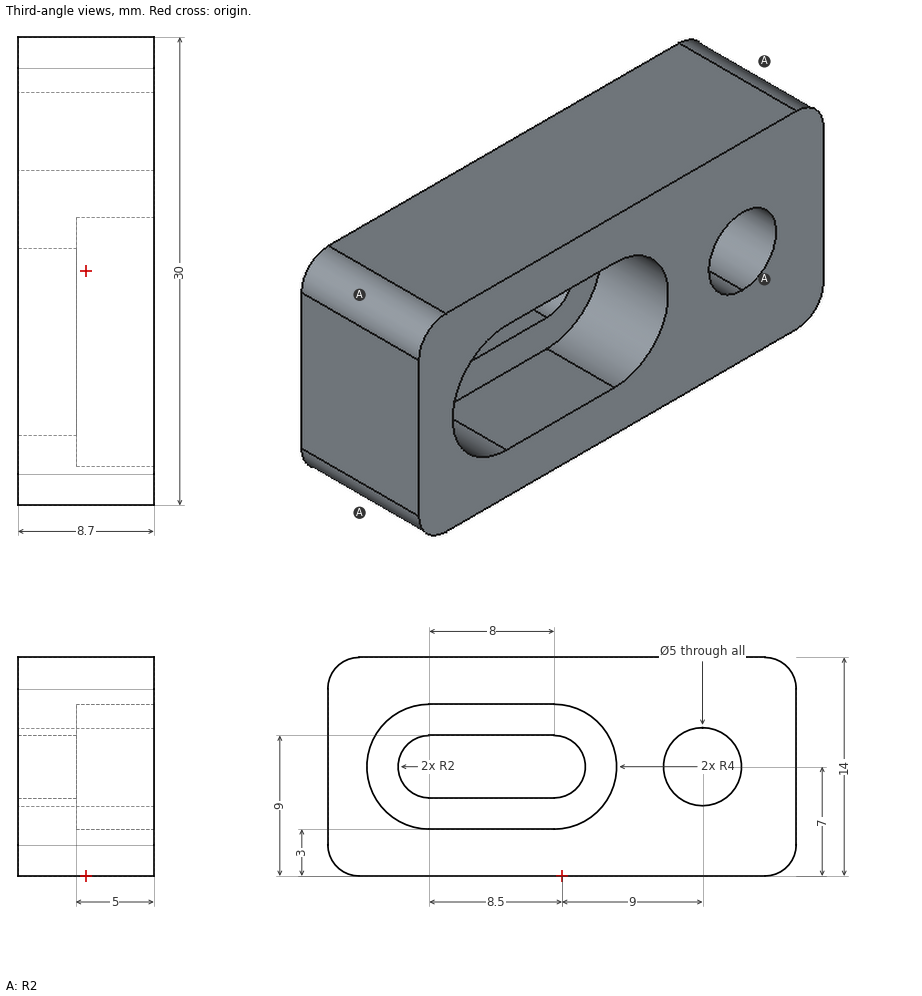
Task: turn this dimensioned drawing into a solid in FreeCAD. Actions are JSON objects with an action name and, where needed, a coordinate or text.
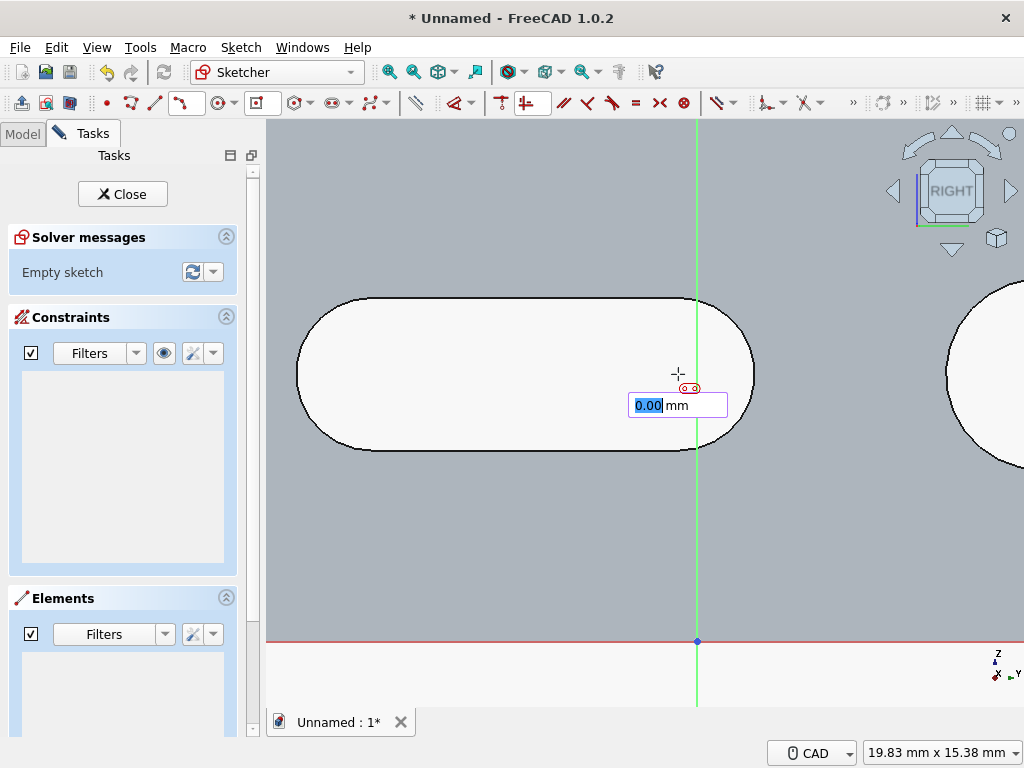
{"action": "left_click", "coordinate": [525, 527]}
{"action": "key", "text": "Escape"}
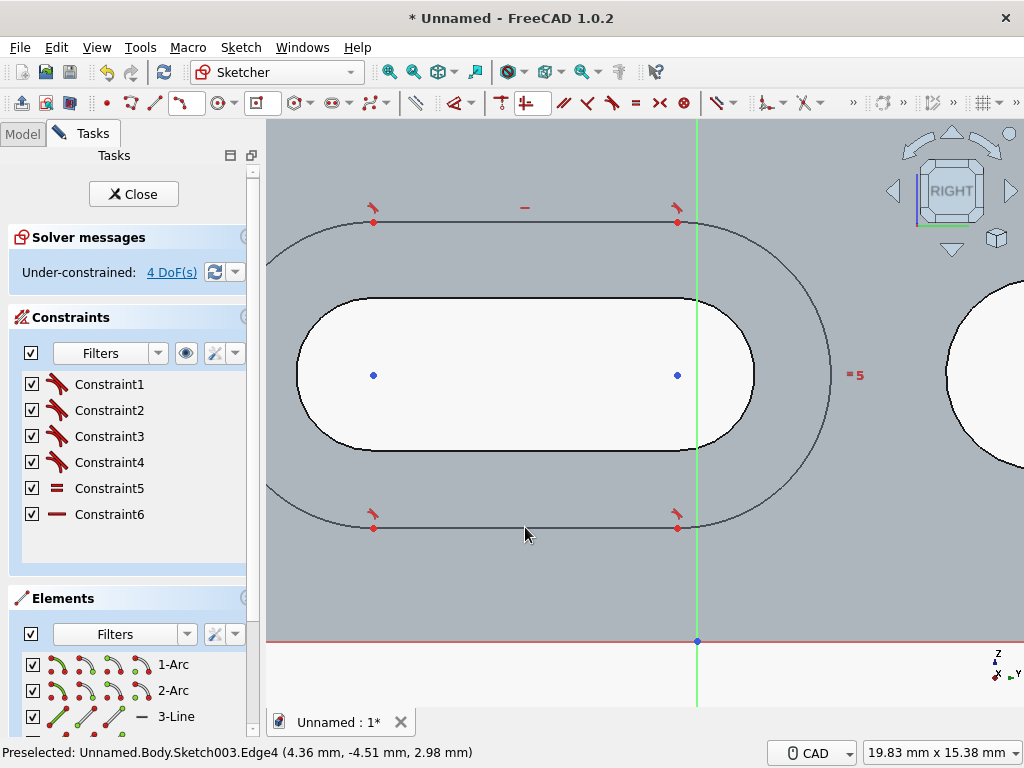
{"action": "left_click", "coordinate": [454, 104]}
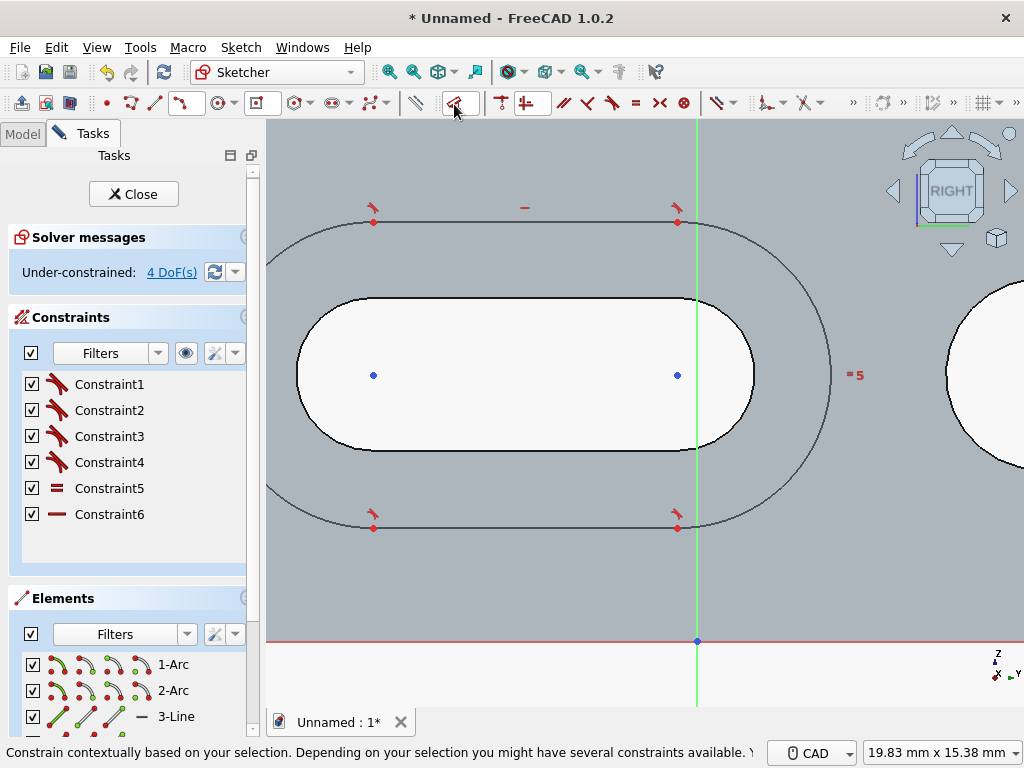
{"action": "scroll", "coordinate": [680, 375], "scroll_direction": "down", "scroll_amount": 2}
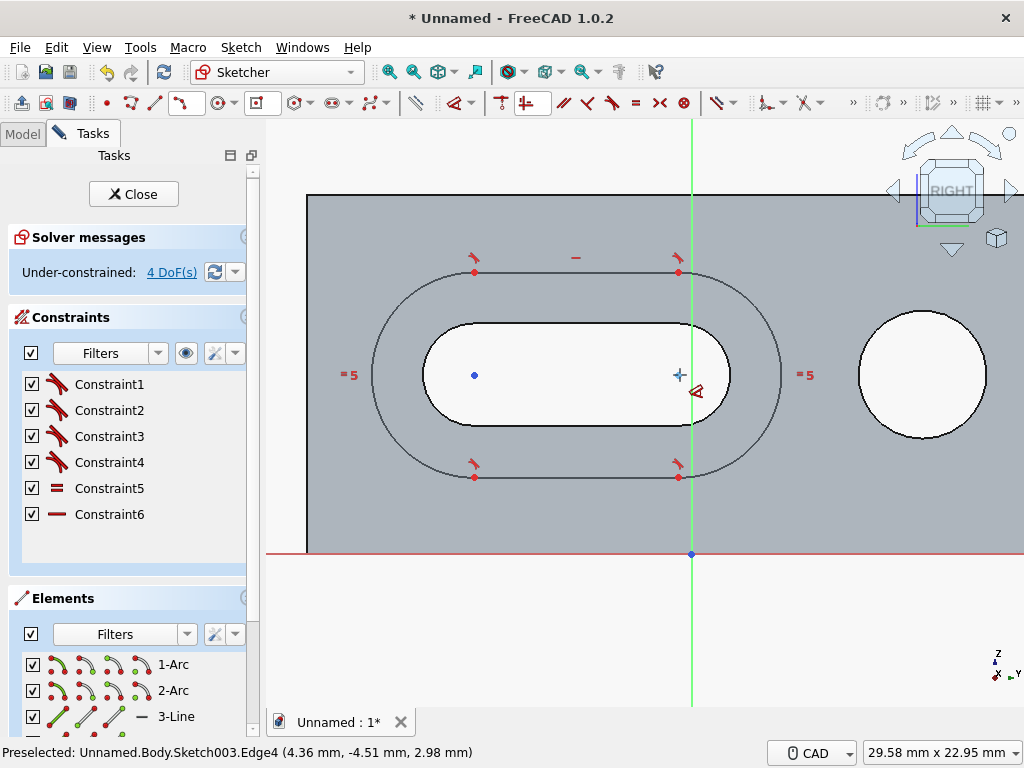
{"action": "left_click", "coordinate": [391, 315]}
{"action": "left_click", "coordinate": [365, 296]}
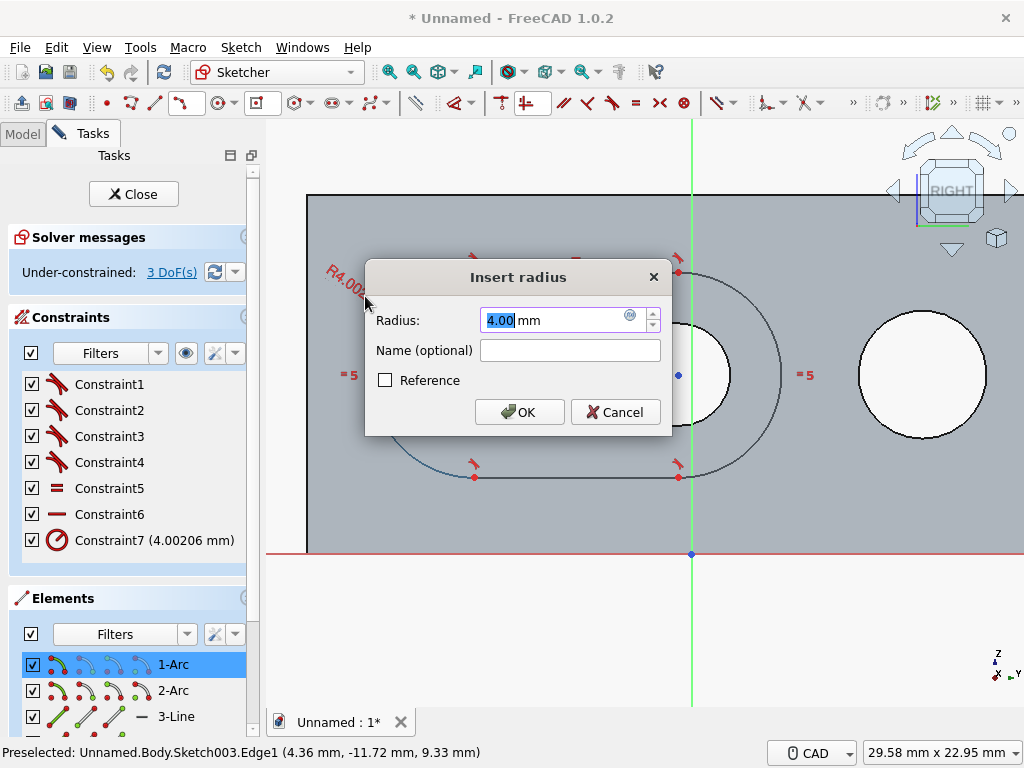
{"action": "type", "text": "4"}
{"action": "key", "text": "Return"}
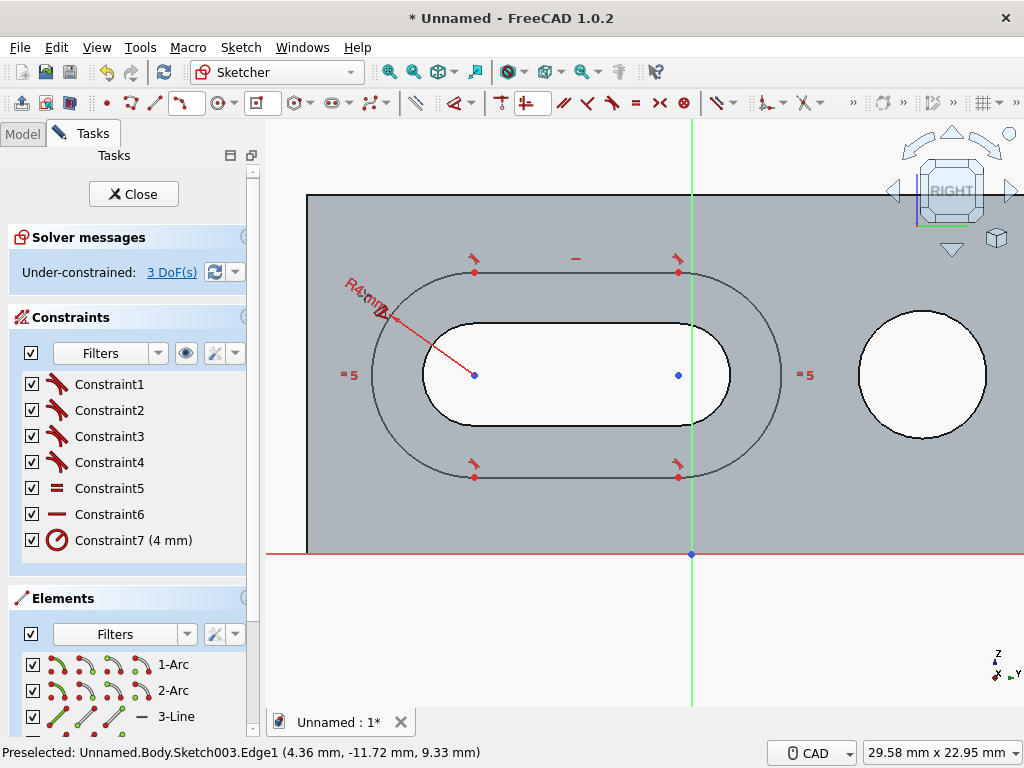
{"action": "left_click", "coordinate": [536, 273]}
{"action": "left_click", "coordinate": [577, 239]}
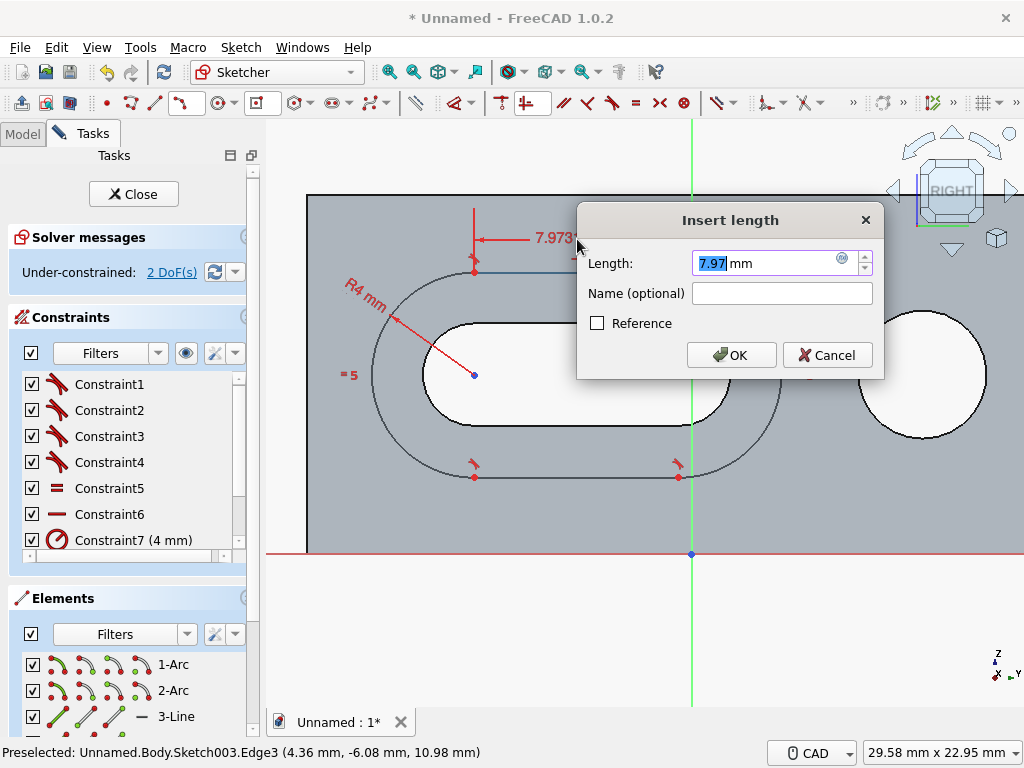
{"action": "type", "text": "8"}
{"action": "key", "text": "Return"}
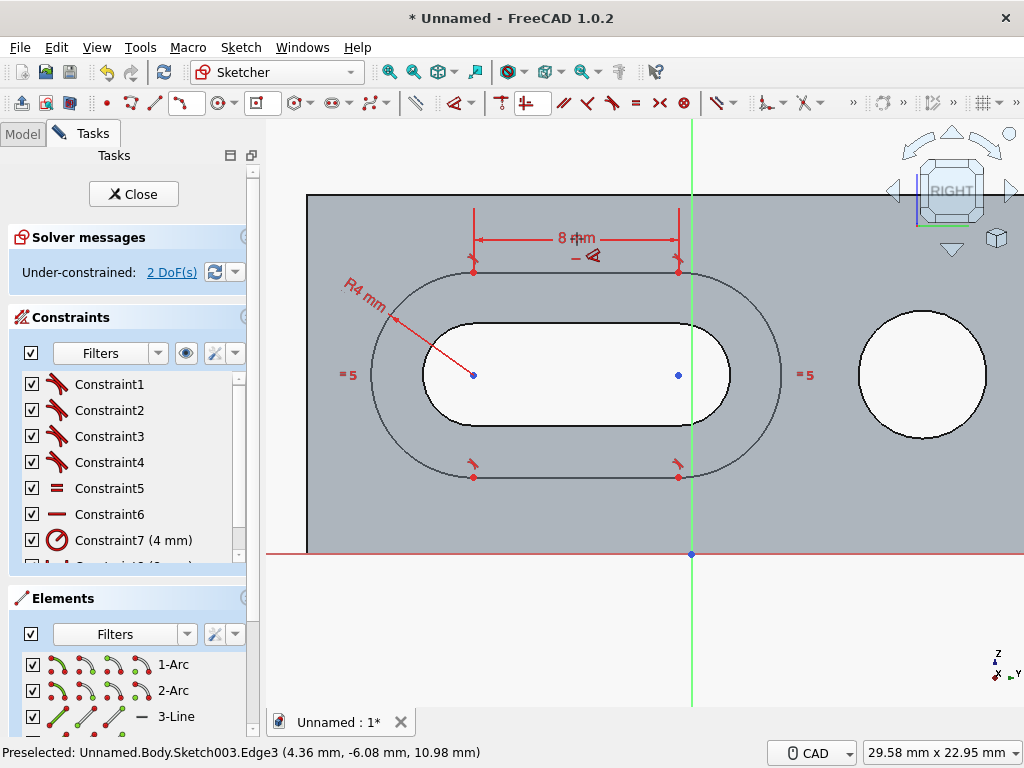
{"action": "left_click", "coordinate": [474, 478]}
{"action": "left_click", "coordinate": [726, 516]}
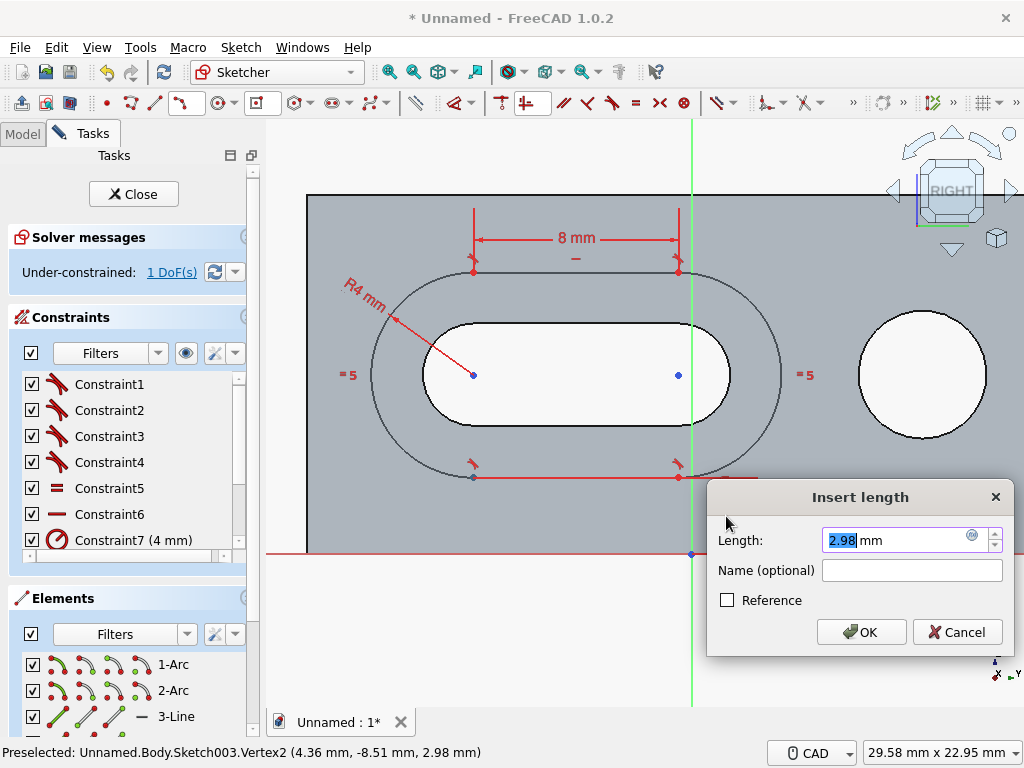
{"action": "type", "text": "3"}
{"action": "key", "text": "Return"}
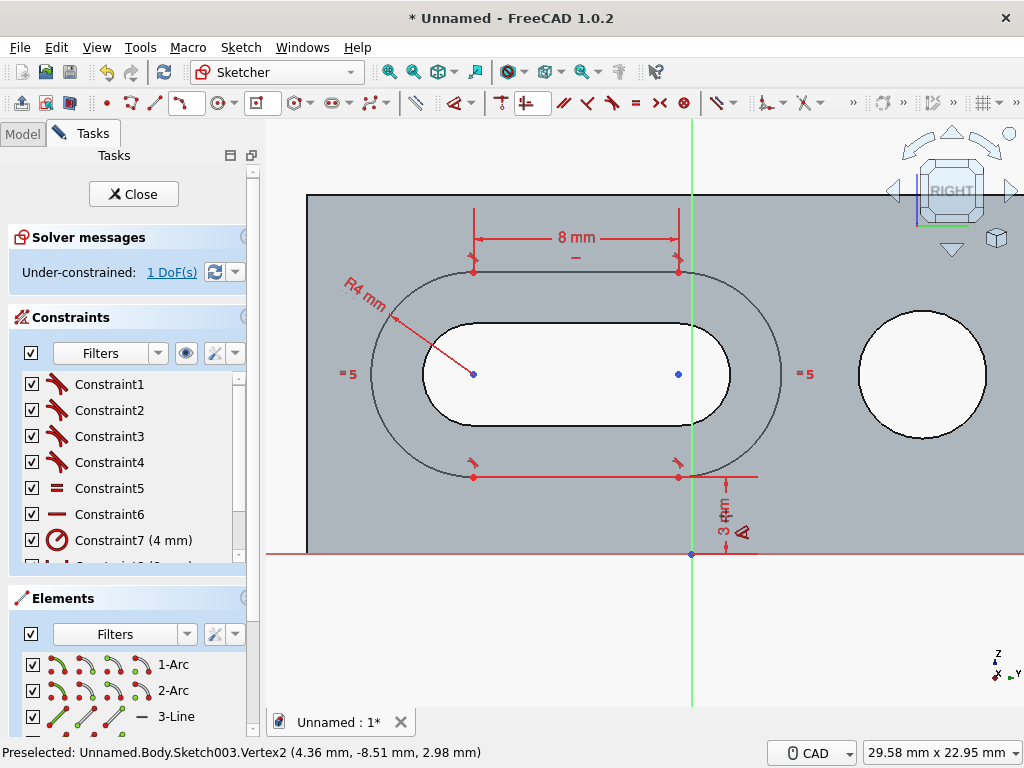
{"action": "left_click", "coordinate": [474, 272]}
{"action": "left_click", "coordinate": [583, 588]}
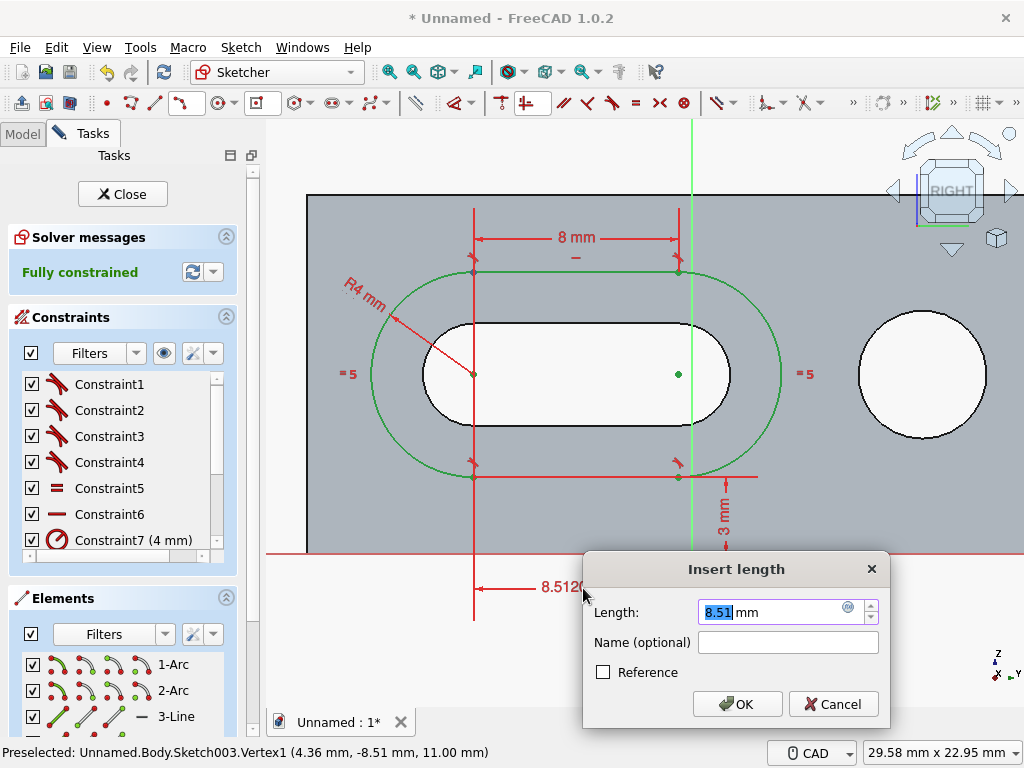
{"action": "type", "text": "8.5"}
{"action": "key", "text": "Return"}
{"action": "key", "text": "Escape"}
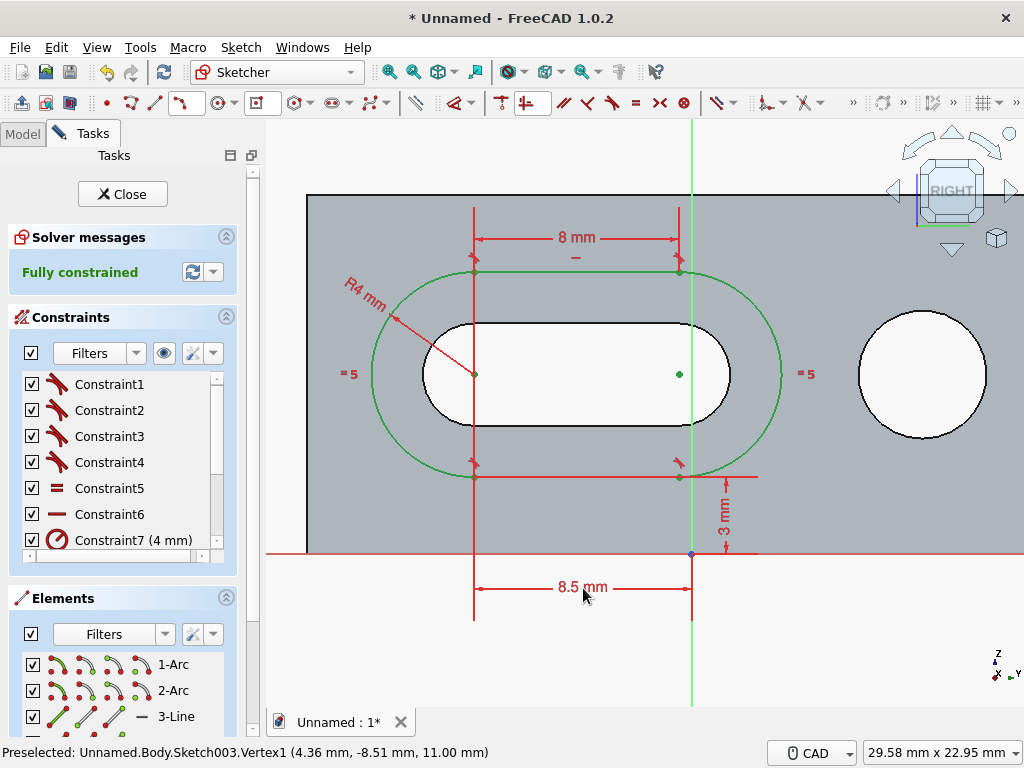
{"action": "left_click", "coordinate": [123, 194]}